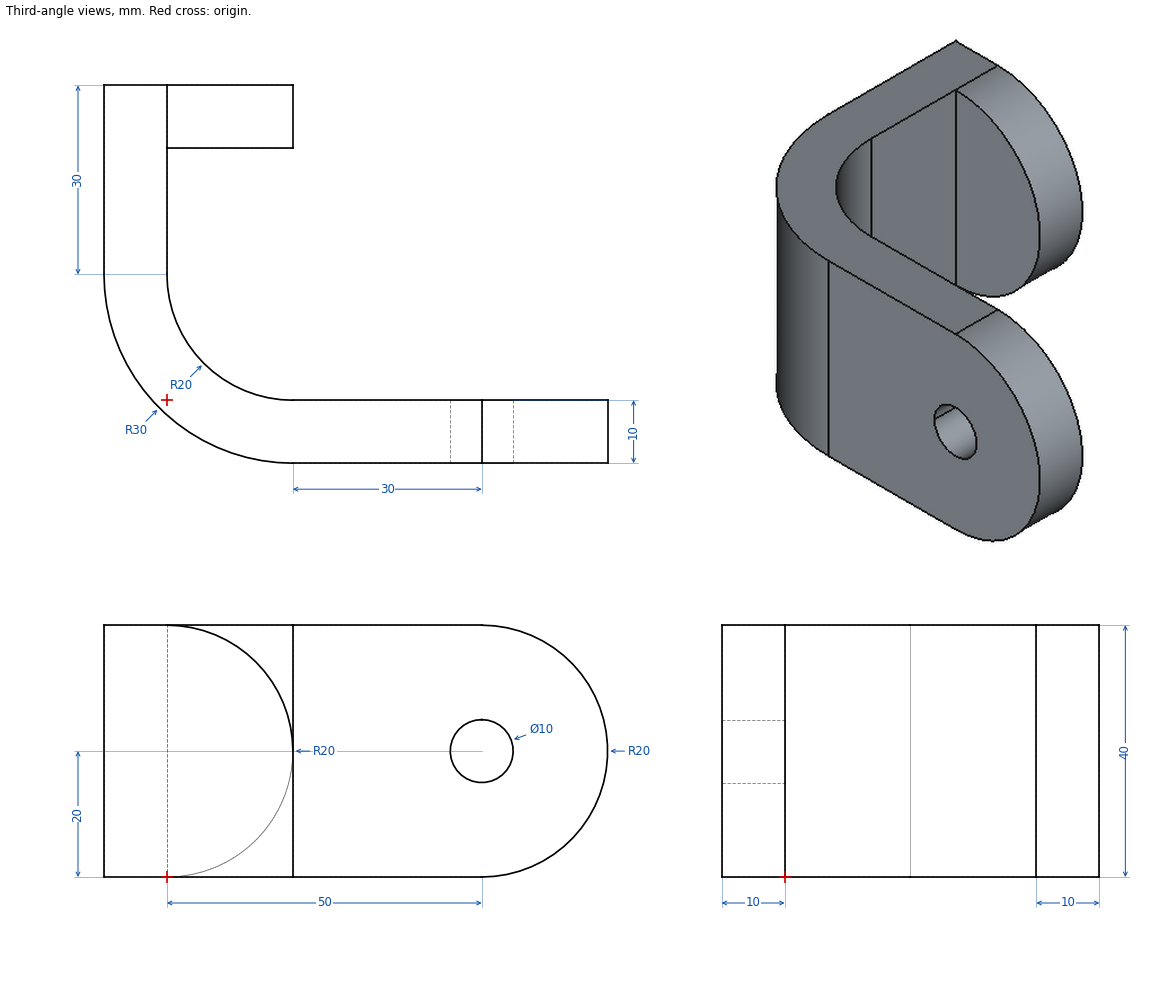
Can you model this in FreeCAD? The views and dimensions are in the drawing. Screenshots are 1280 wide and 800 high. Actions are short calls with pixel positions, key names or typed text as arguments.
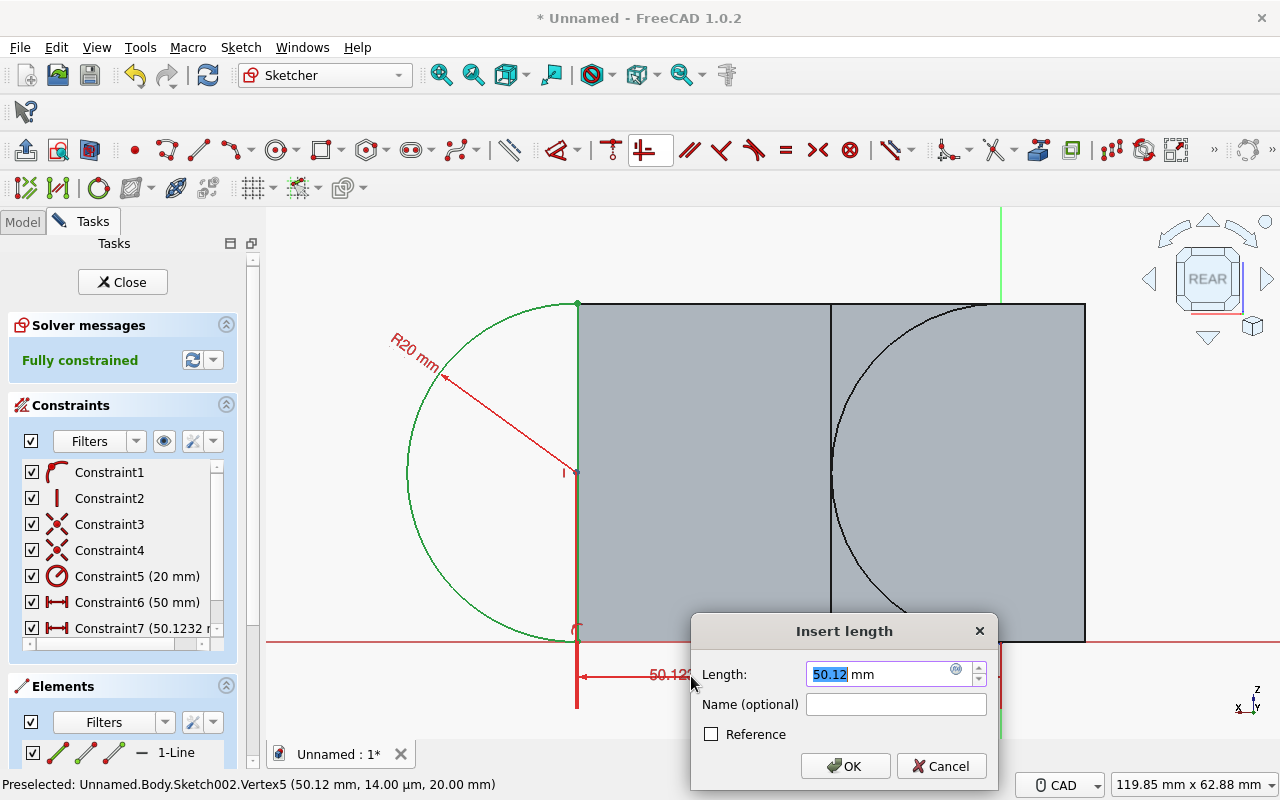
text(50)
key(Return)
key(Escape)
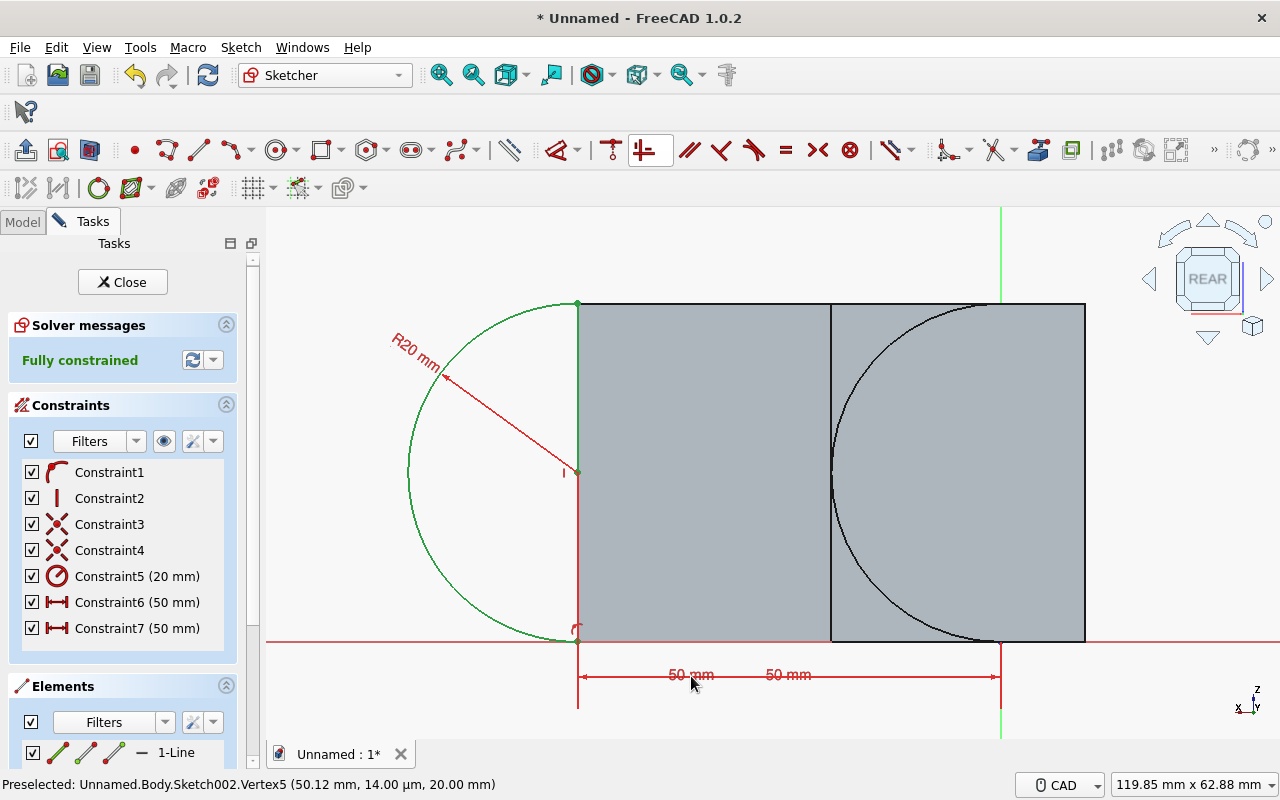
click(123, 282)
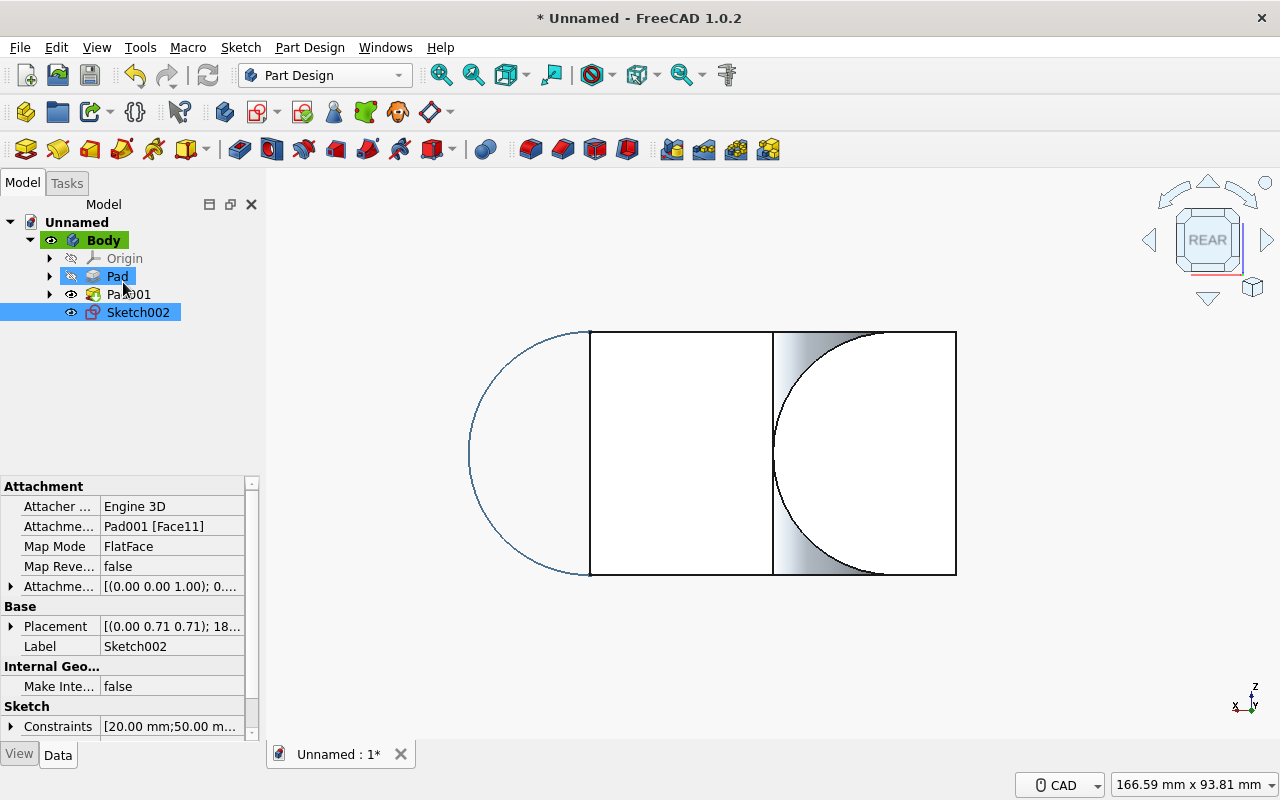
click(26, 150)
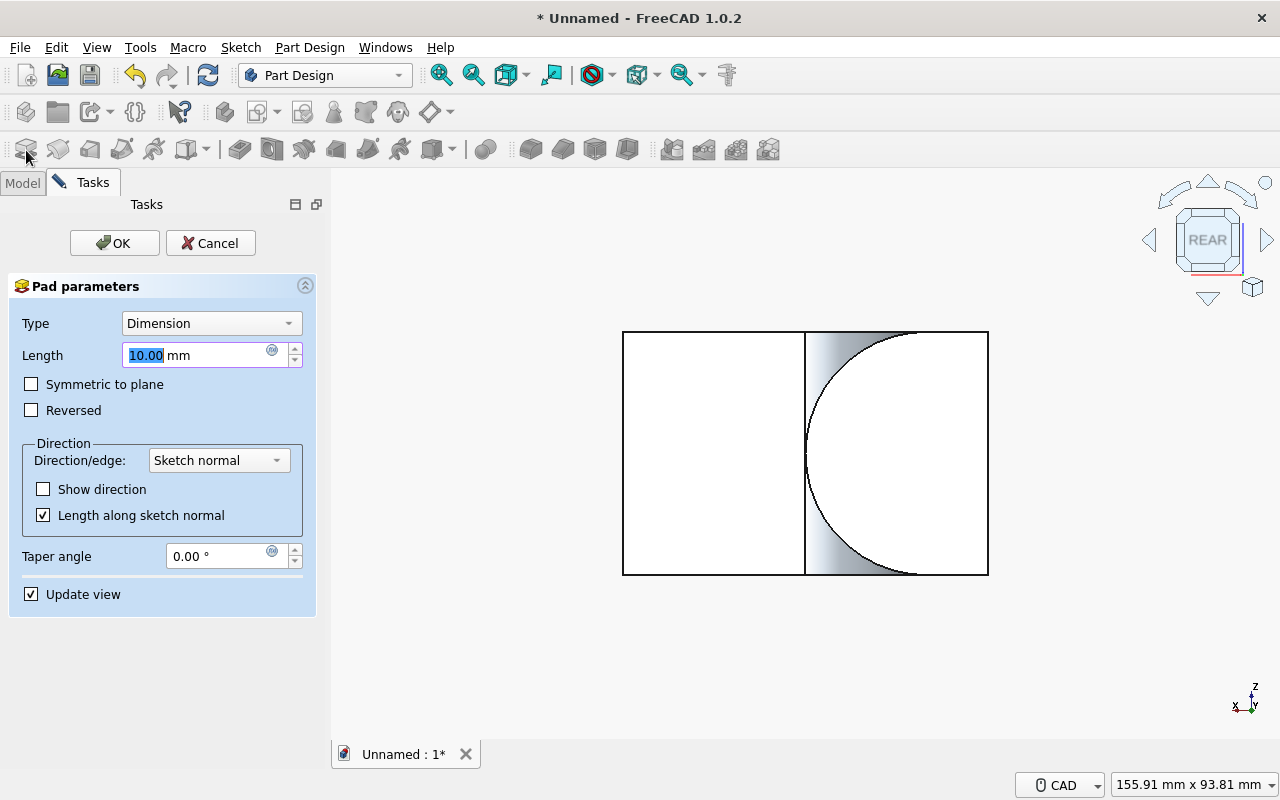
text(10)
key(Tab)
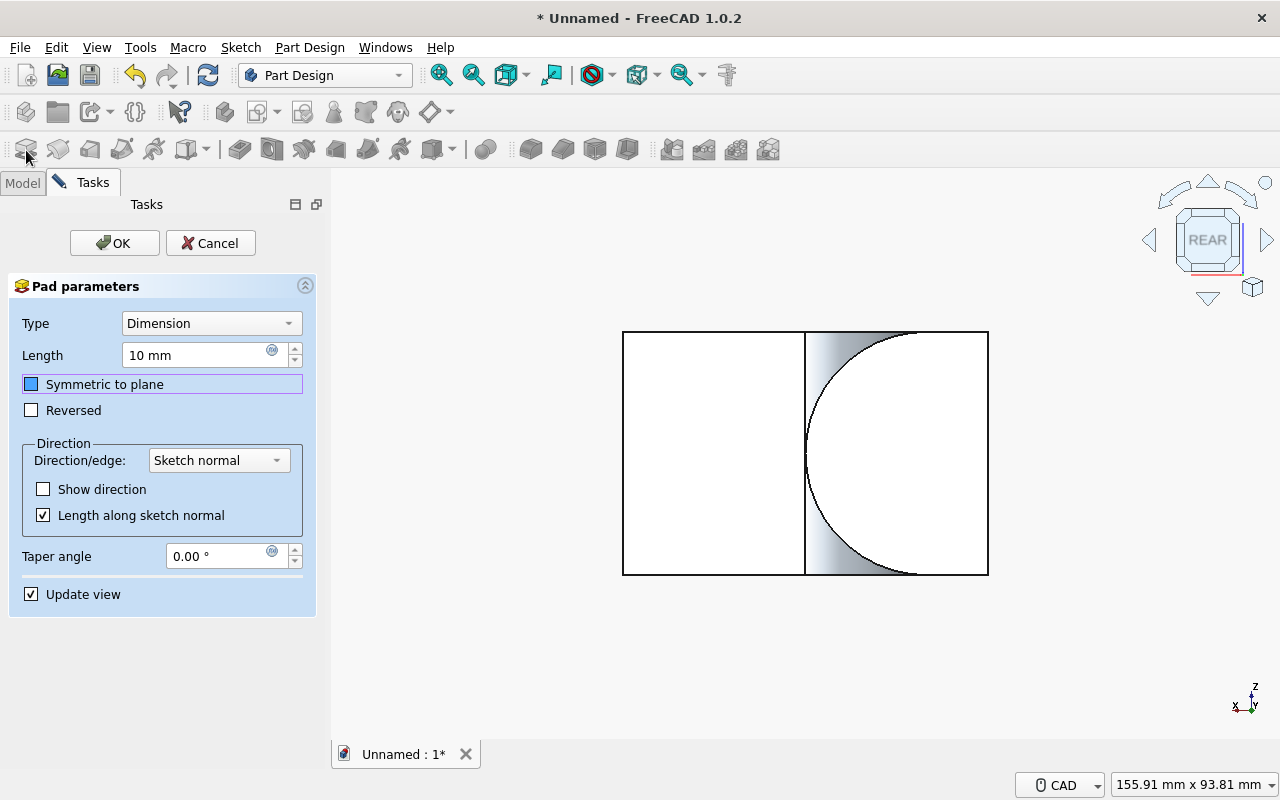
click(30, 410)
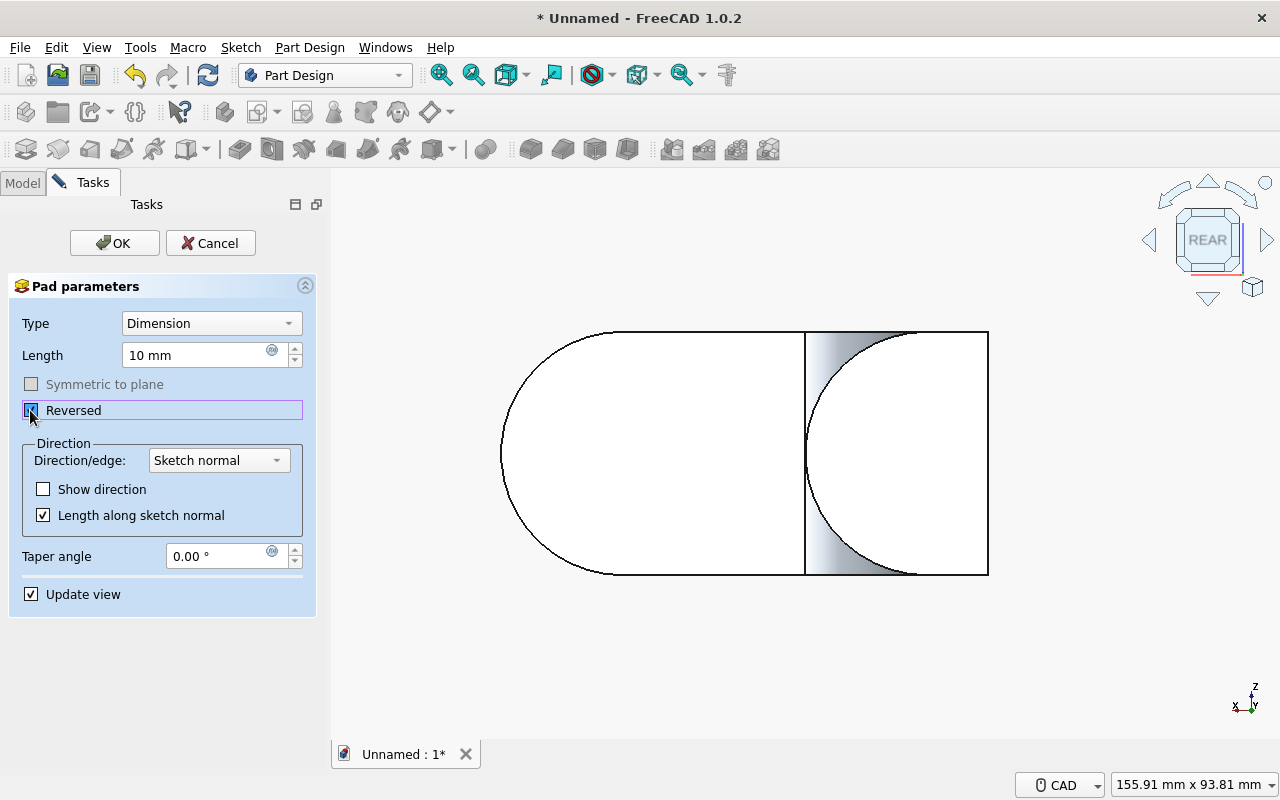
click(115, 243)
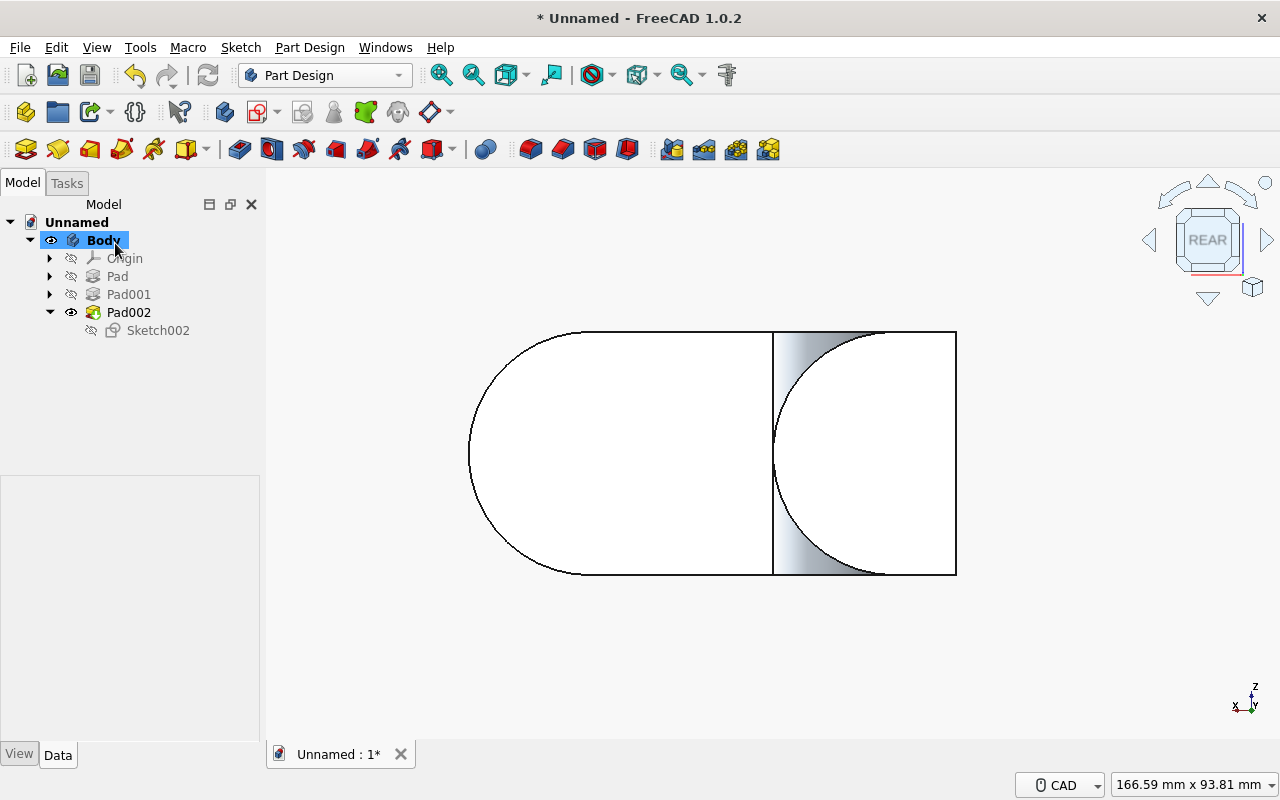
click(621, 452)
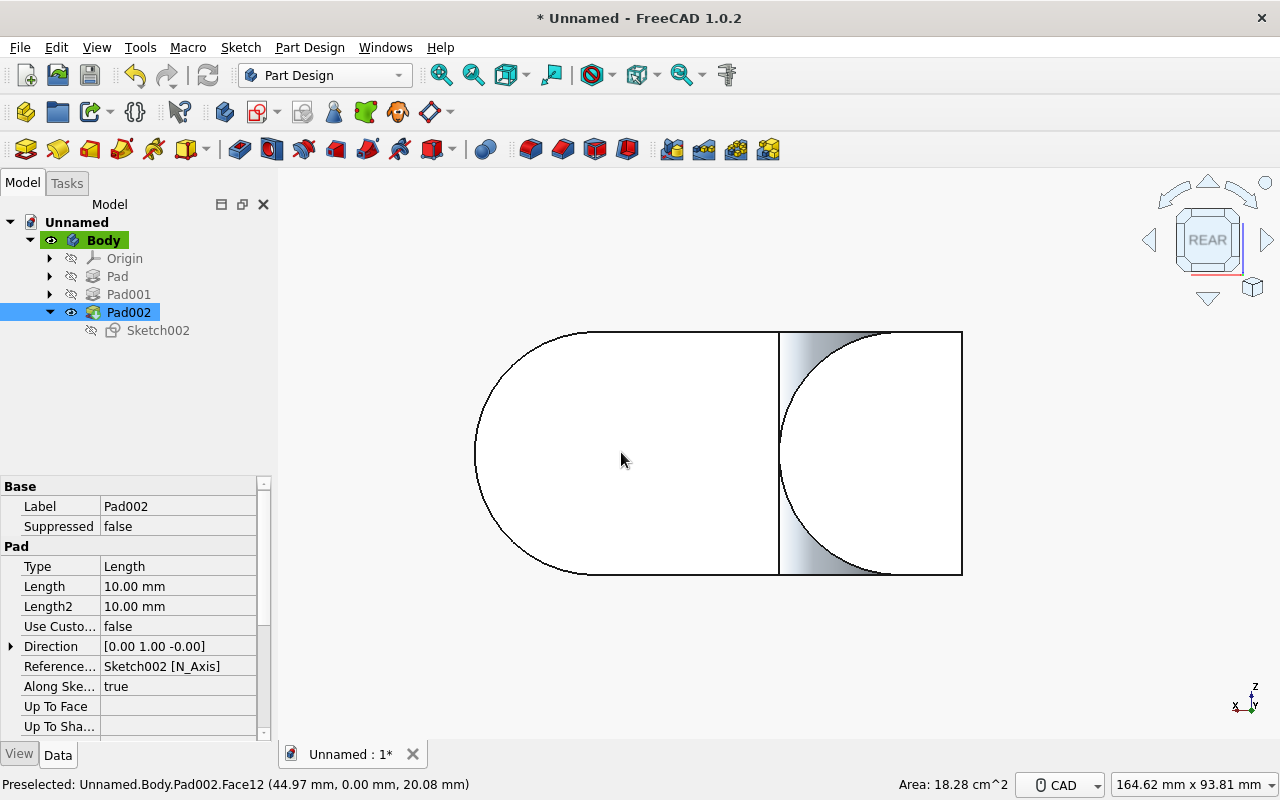
click(258, 112)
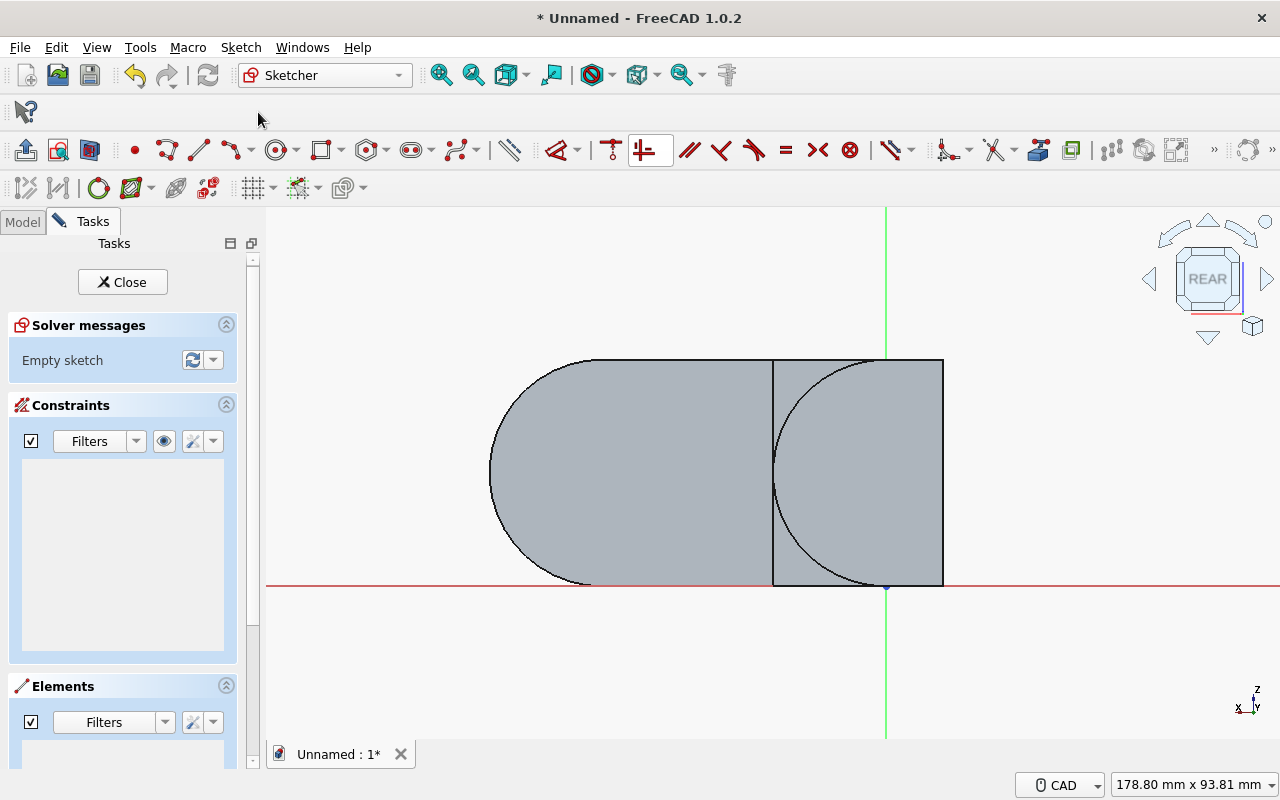
click(90, 150)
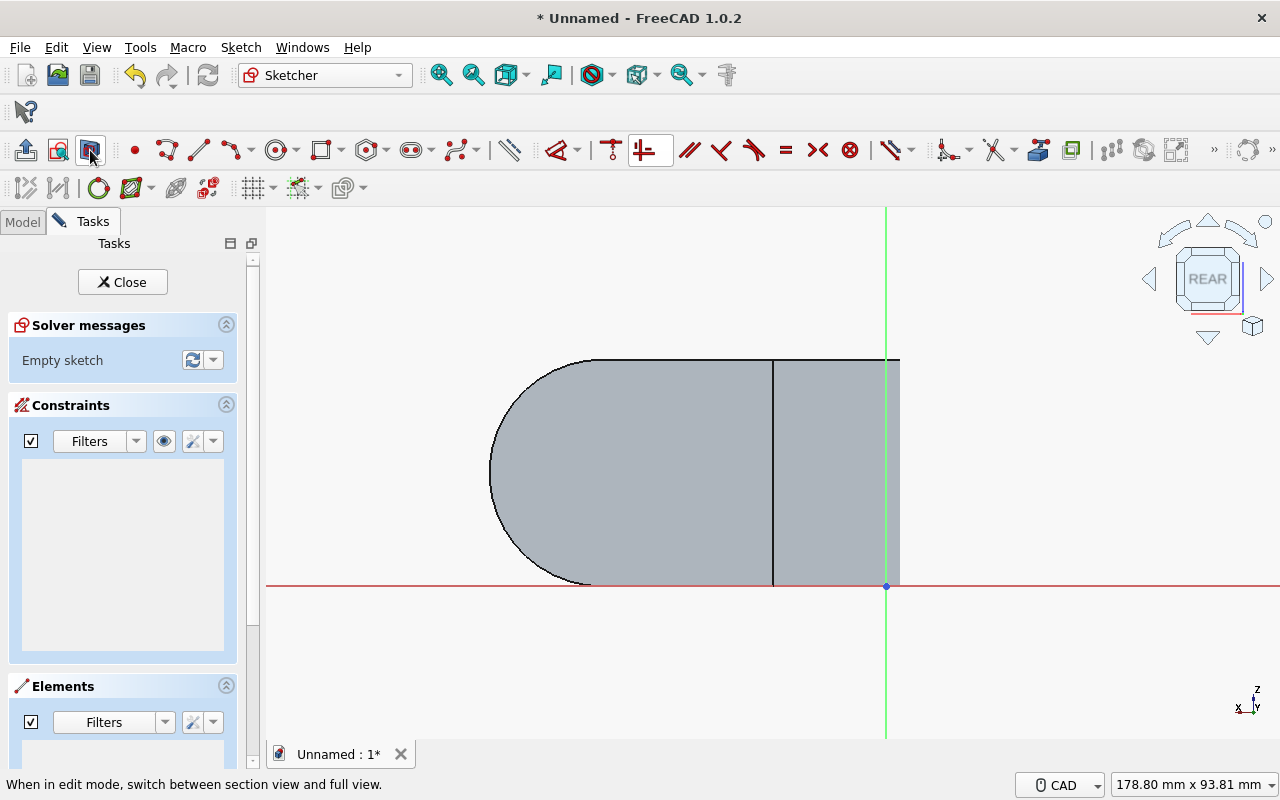
scroll(583, 473, up, 9)